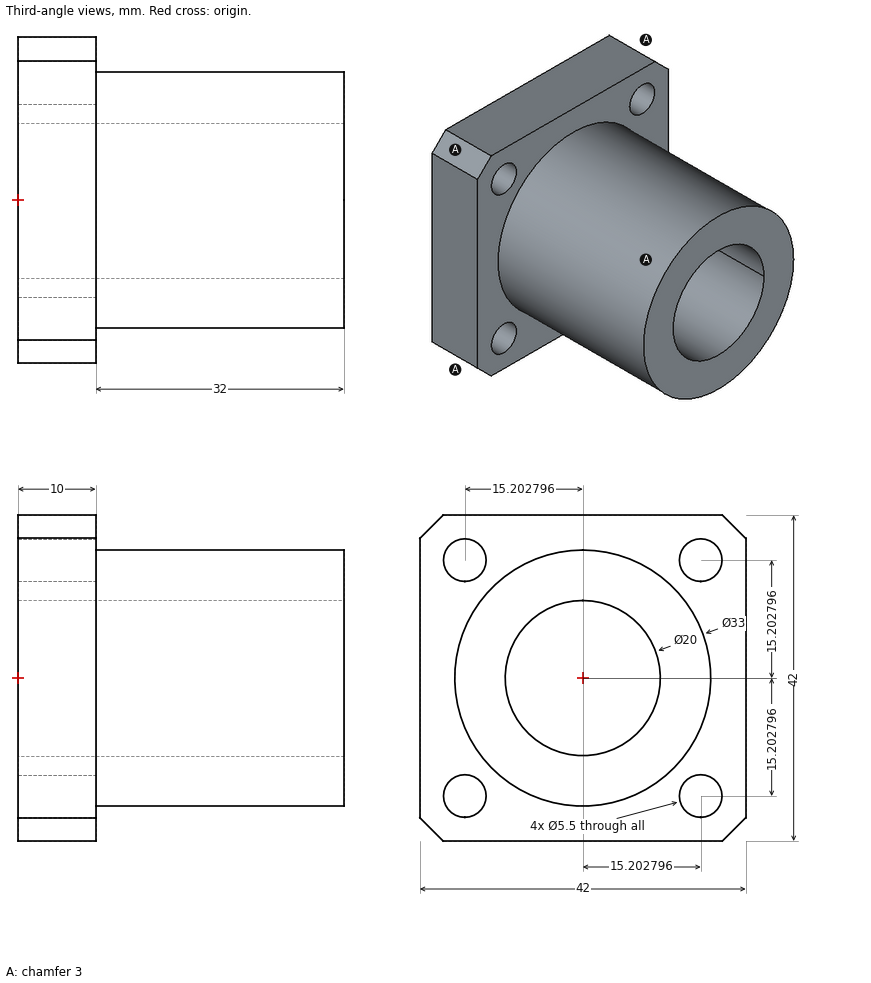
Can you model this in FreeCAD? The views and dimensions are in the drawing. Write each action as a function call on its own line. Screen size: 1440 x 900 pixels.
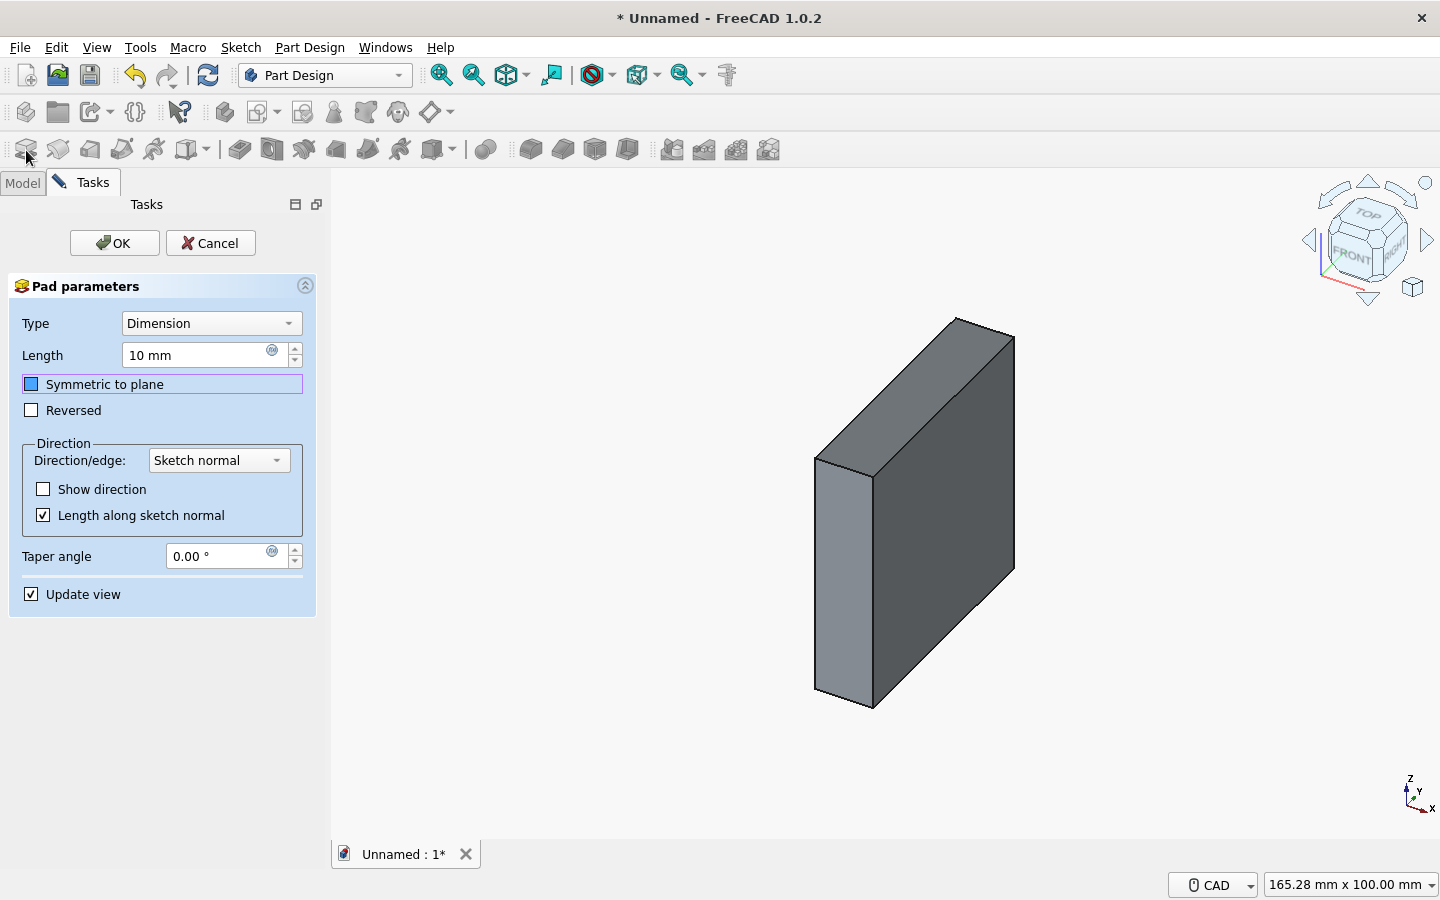
click(115, 243)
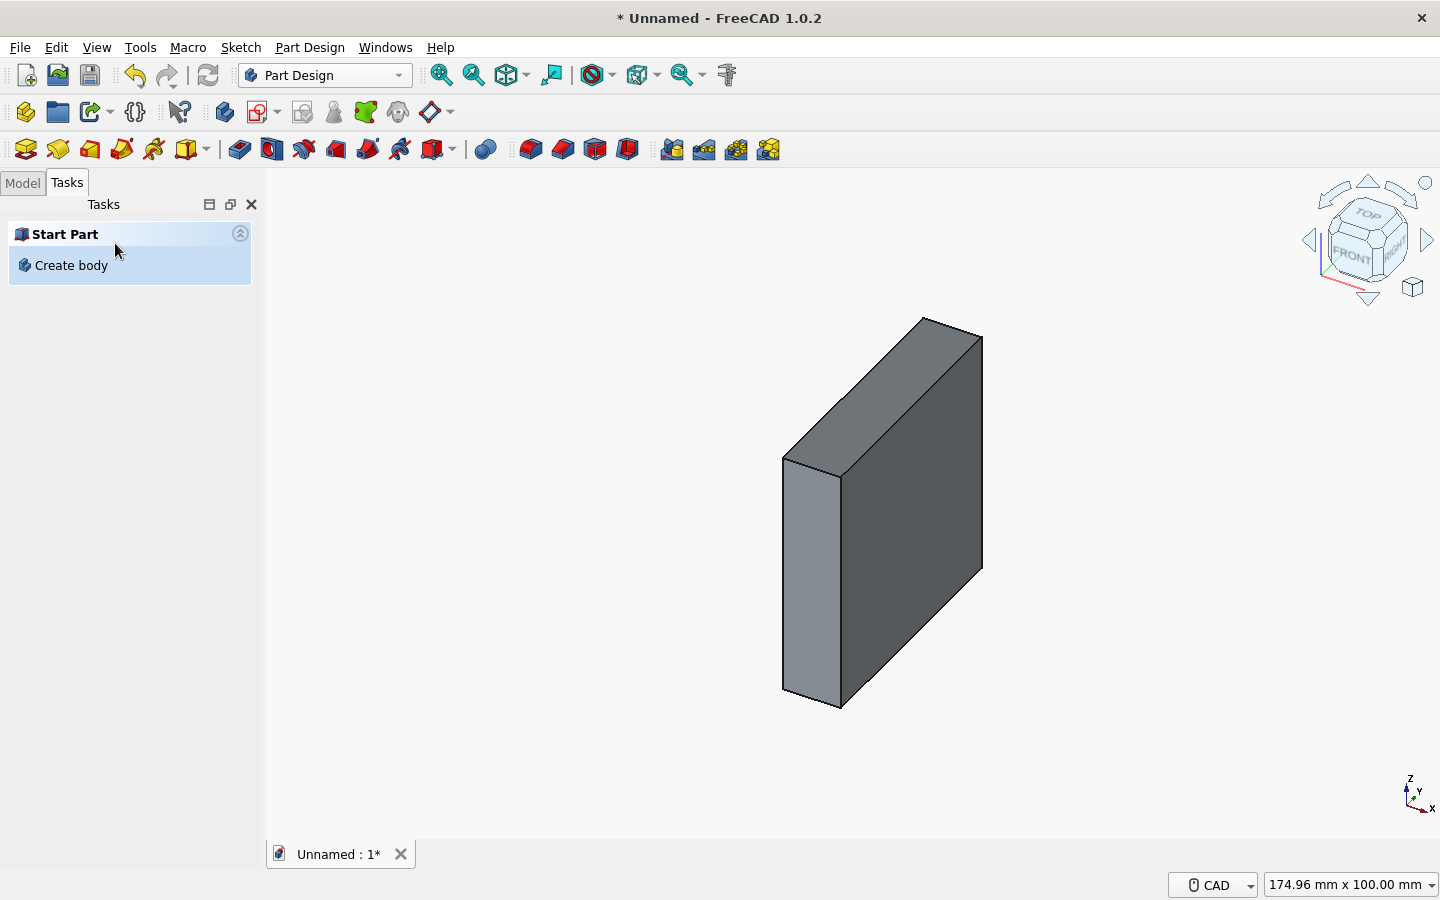
click(911, 522)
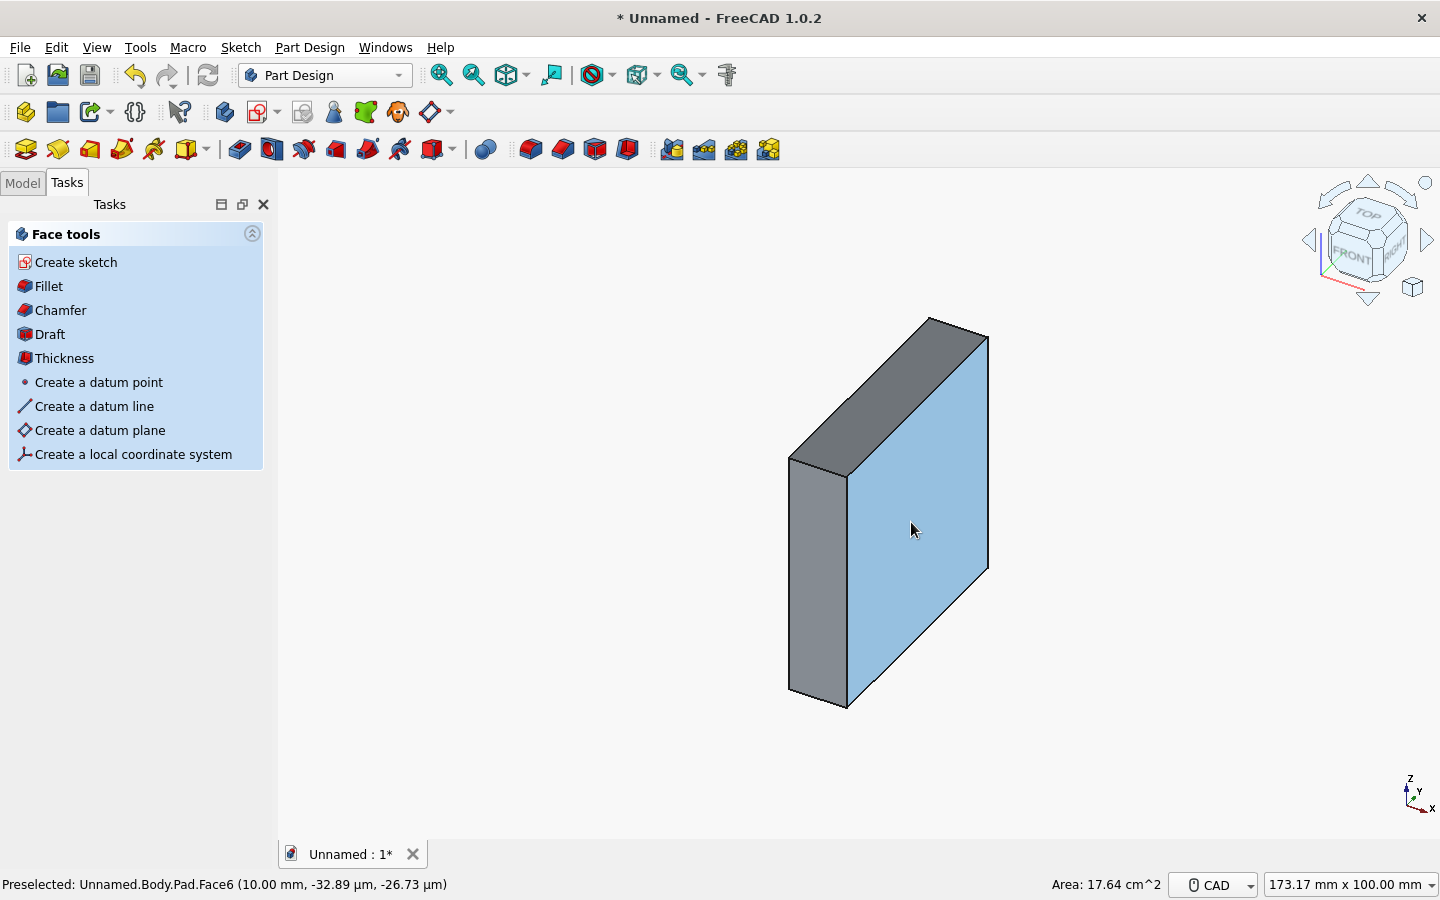
click(258, 112)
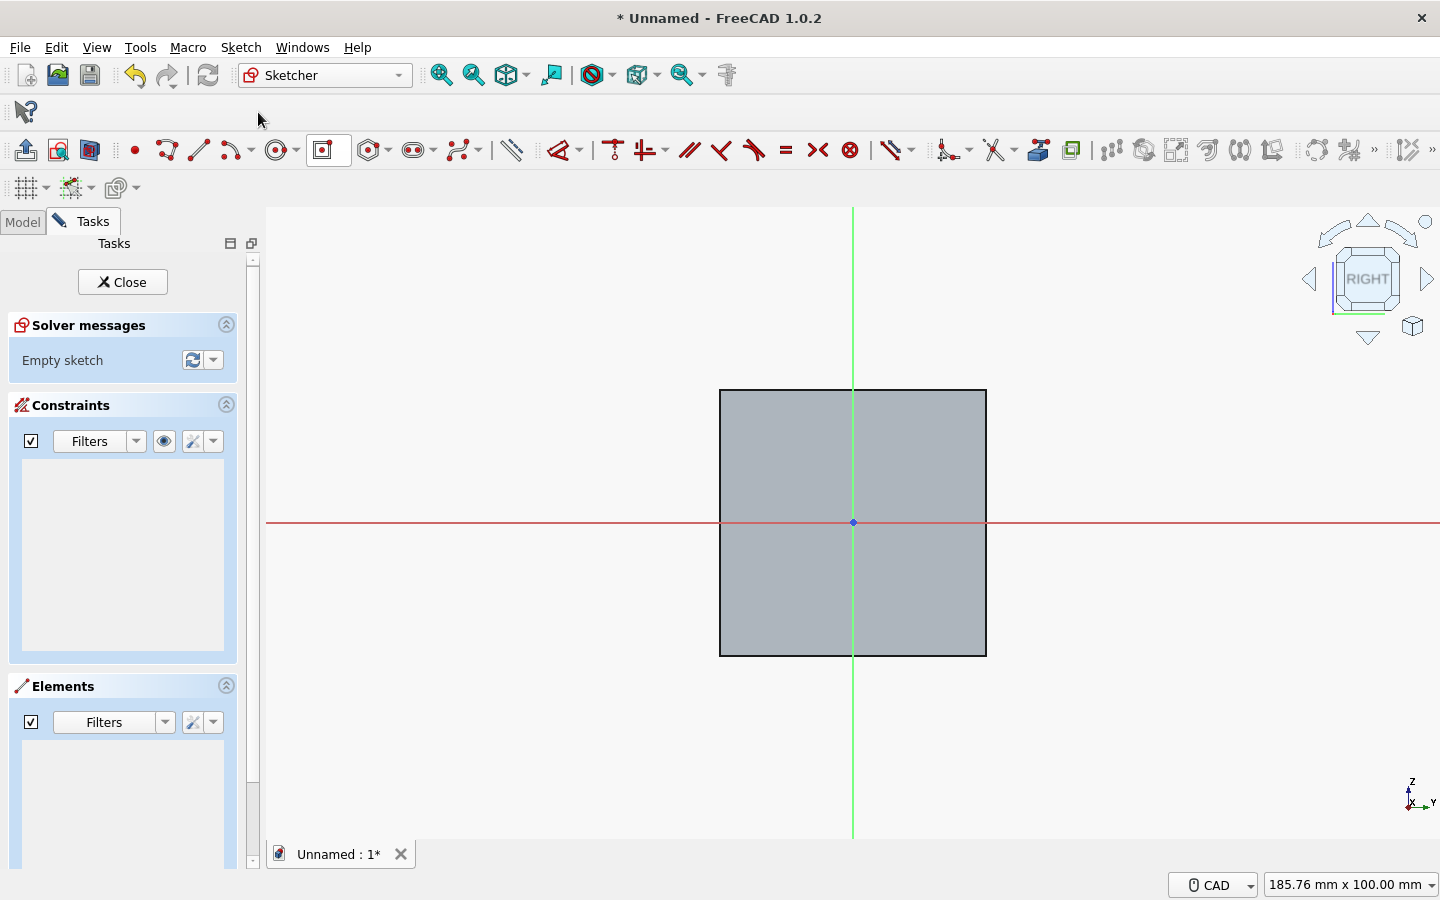
scroll(936, 523, up, 3)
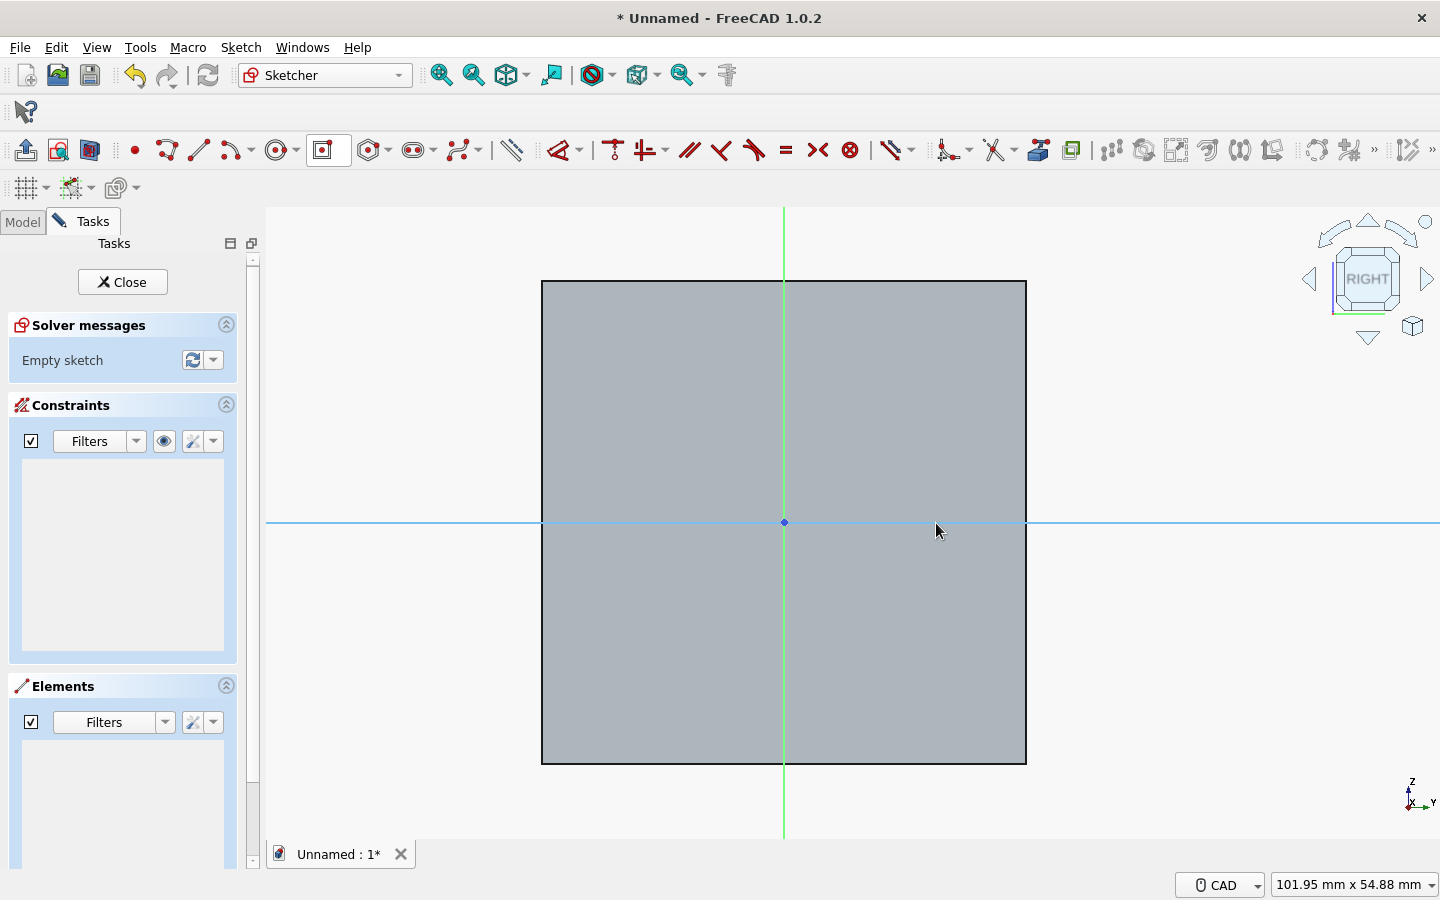
click(276, 150)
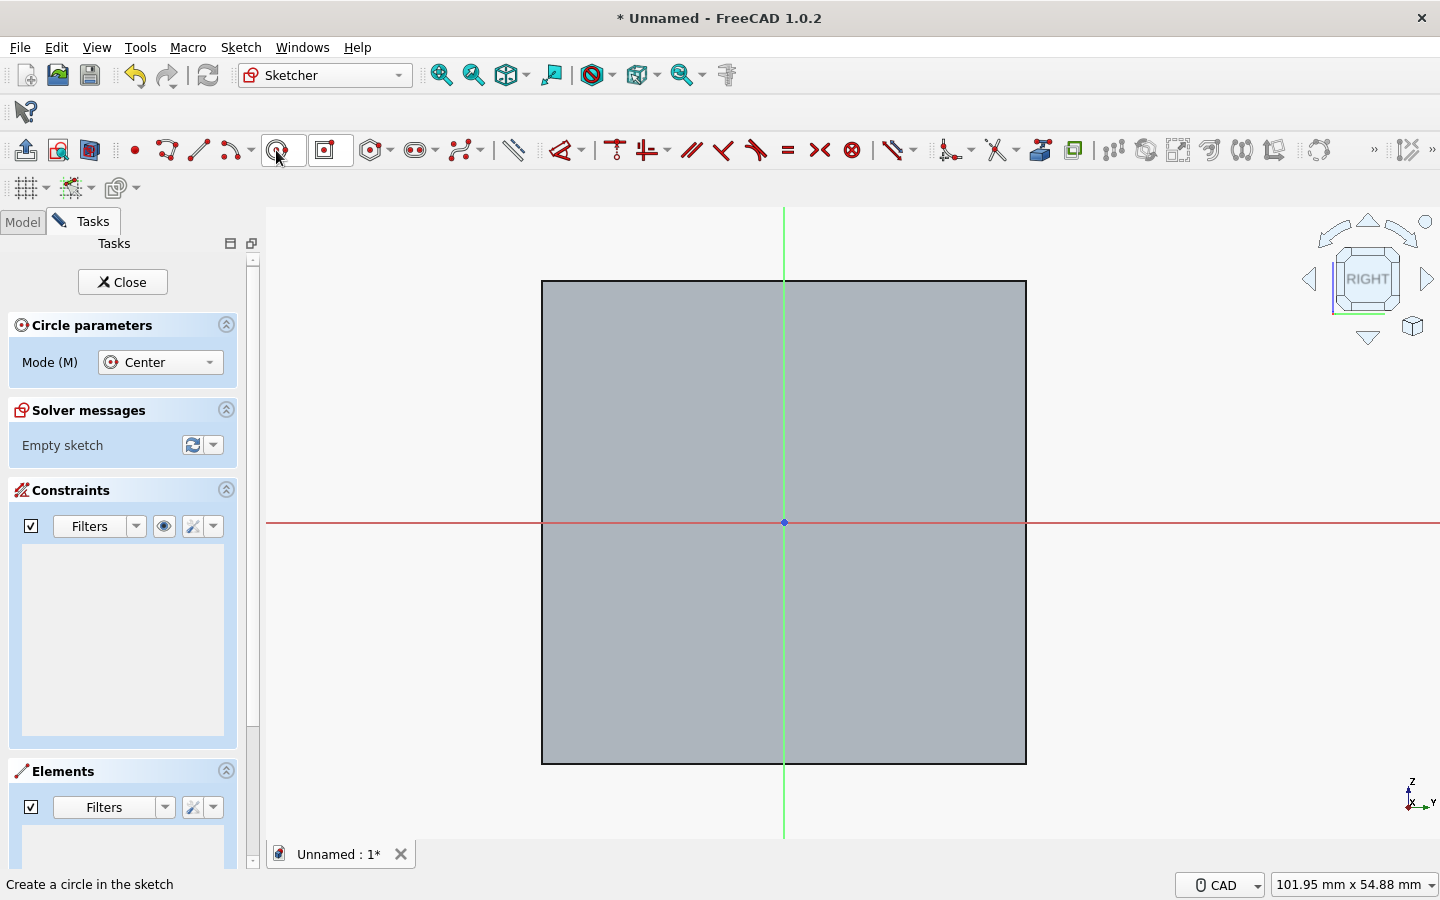
click(784, 523)
click(919, 388)
key(Escape)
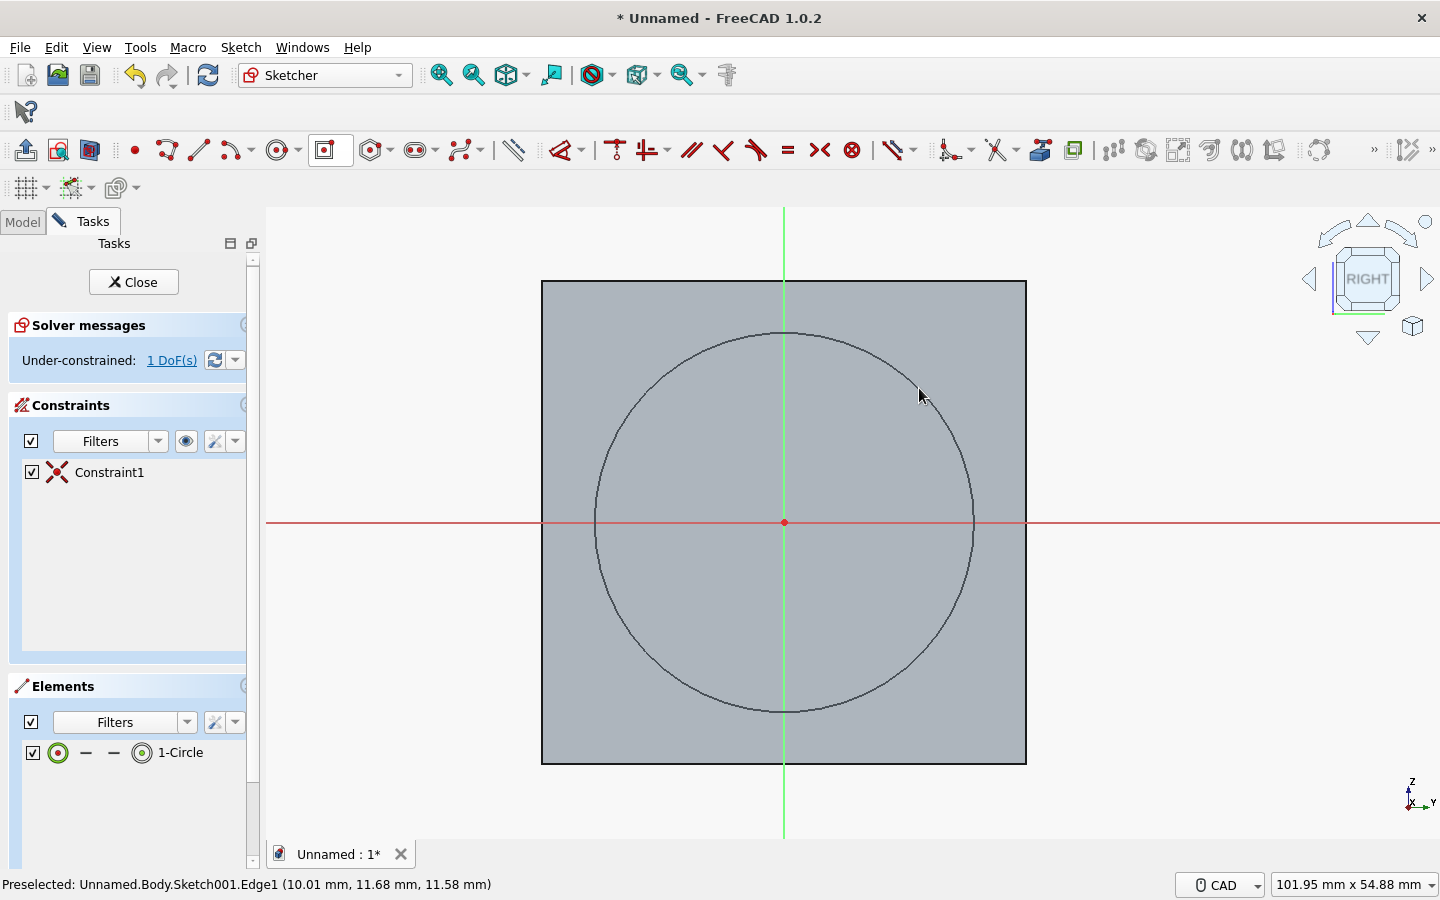
click(560, 150)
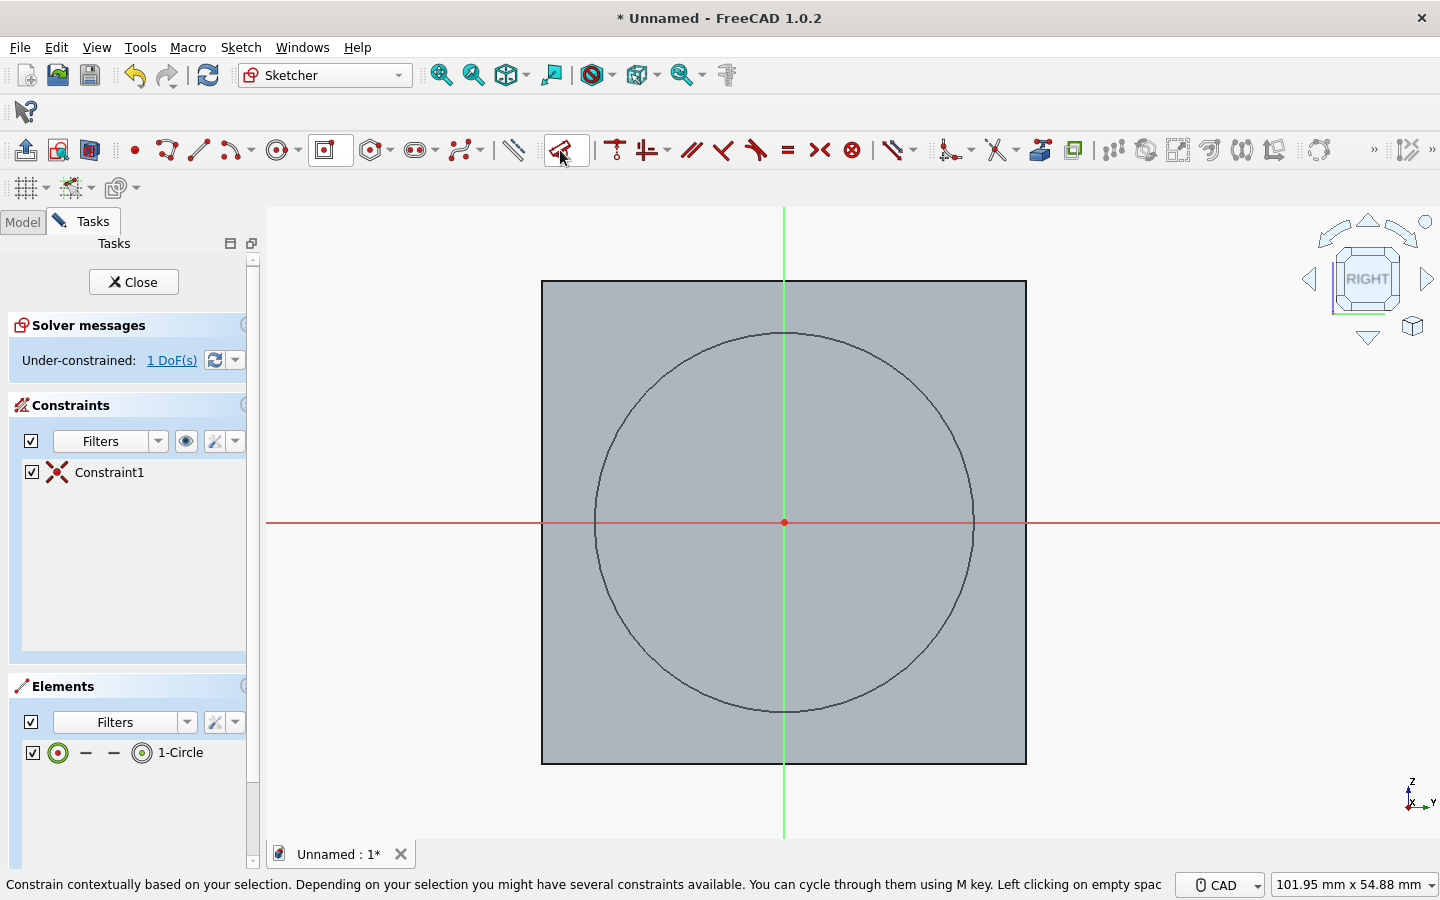
click(918, 388)
click(941, 365)